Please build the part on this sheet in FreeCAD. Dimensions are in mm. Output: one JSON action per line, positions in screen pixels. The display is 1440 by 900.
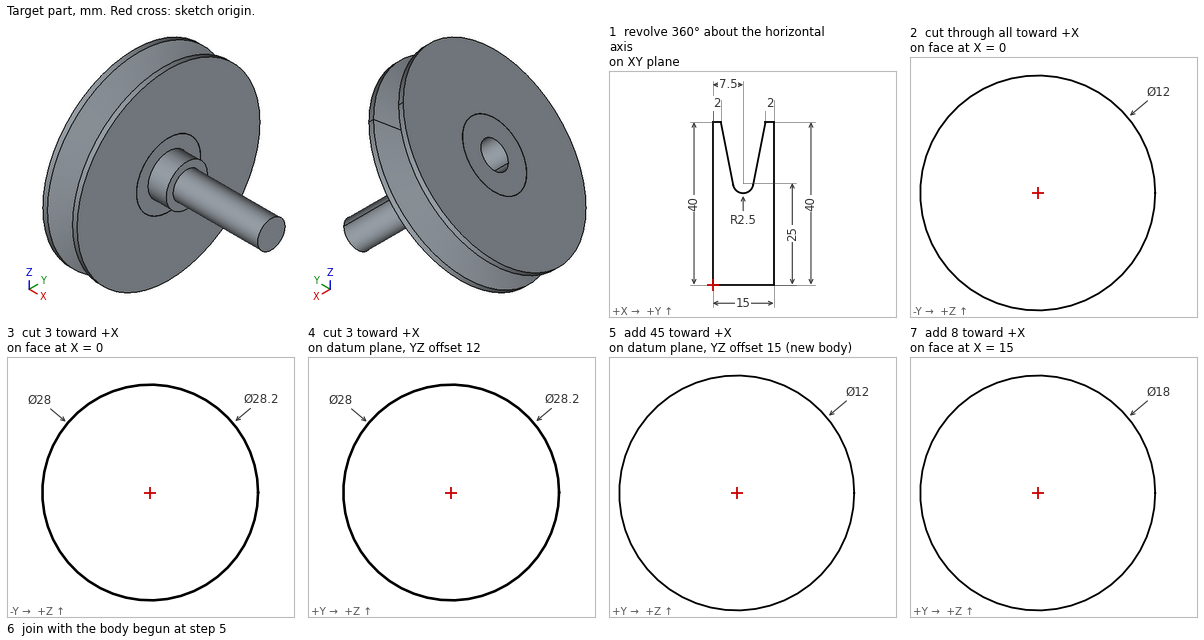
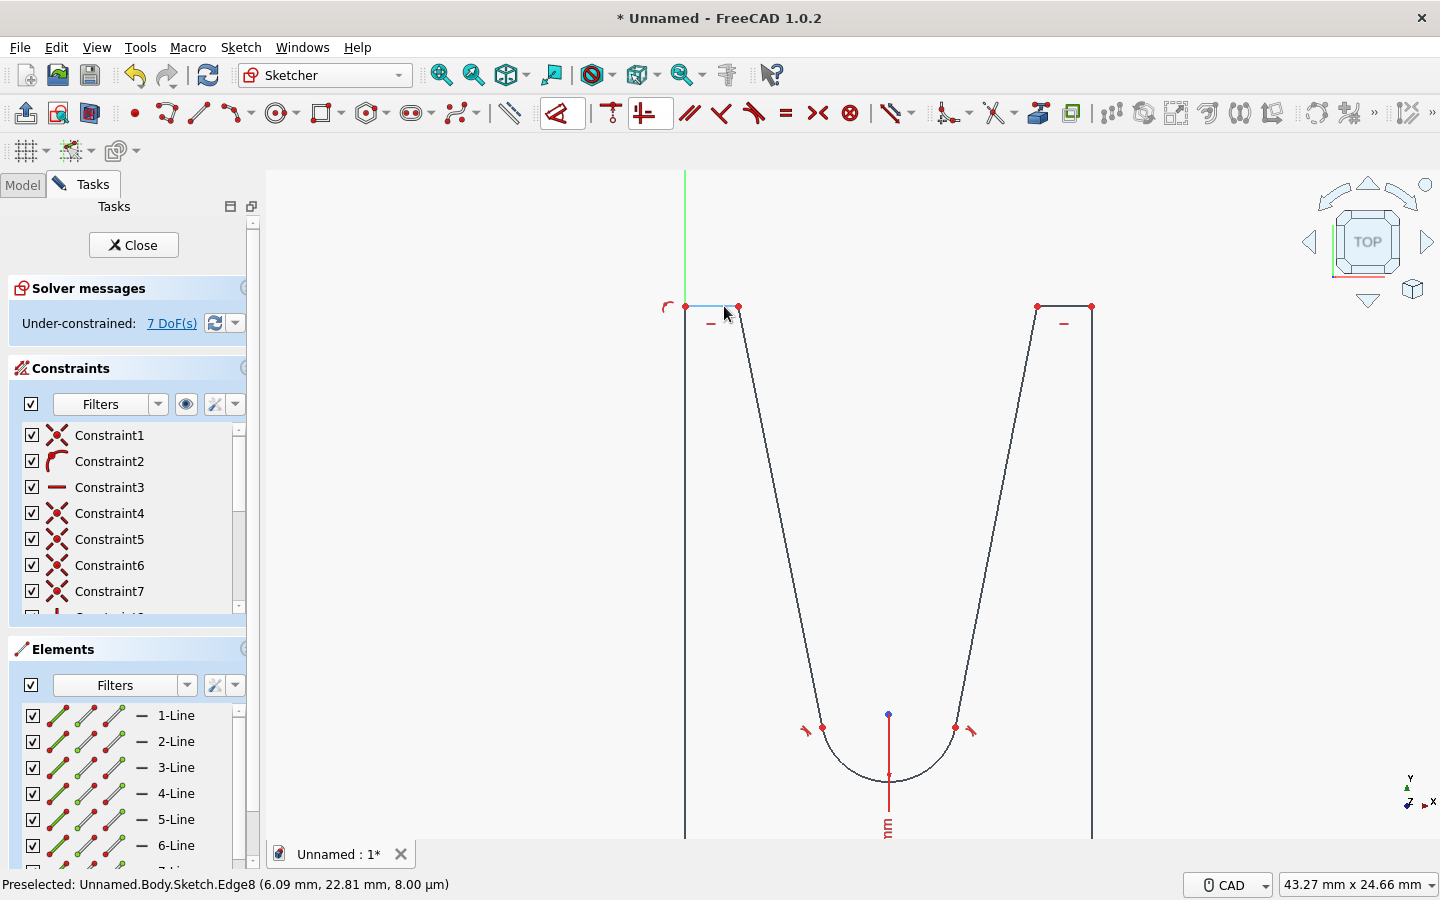
{"action": "left_click", "coordinate": [722, 306]}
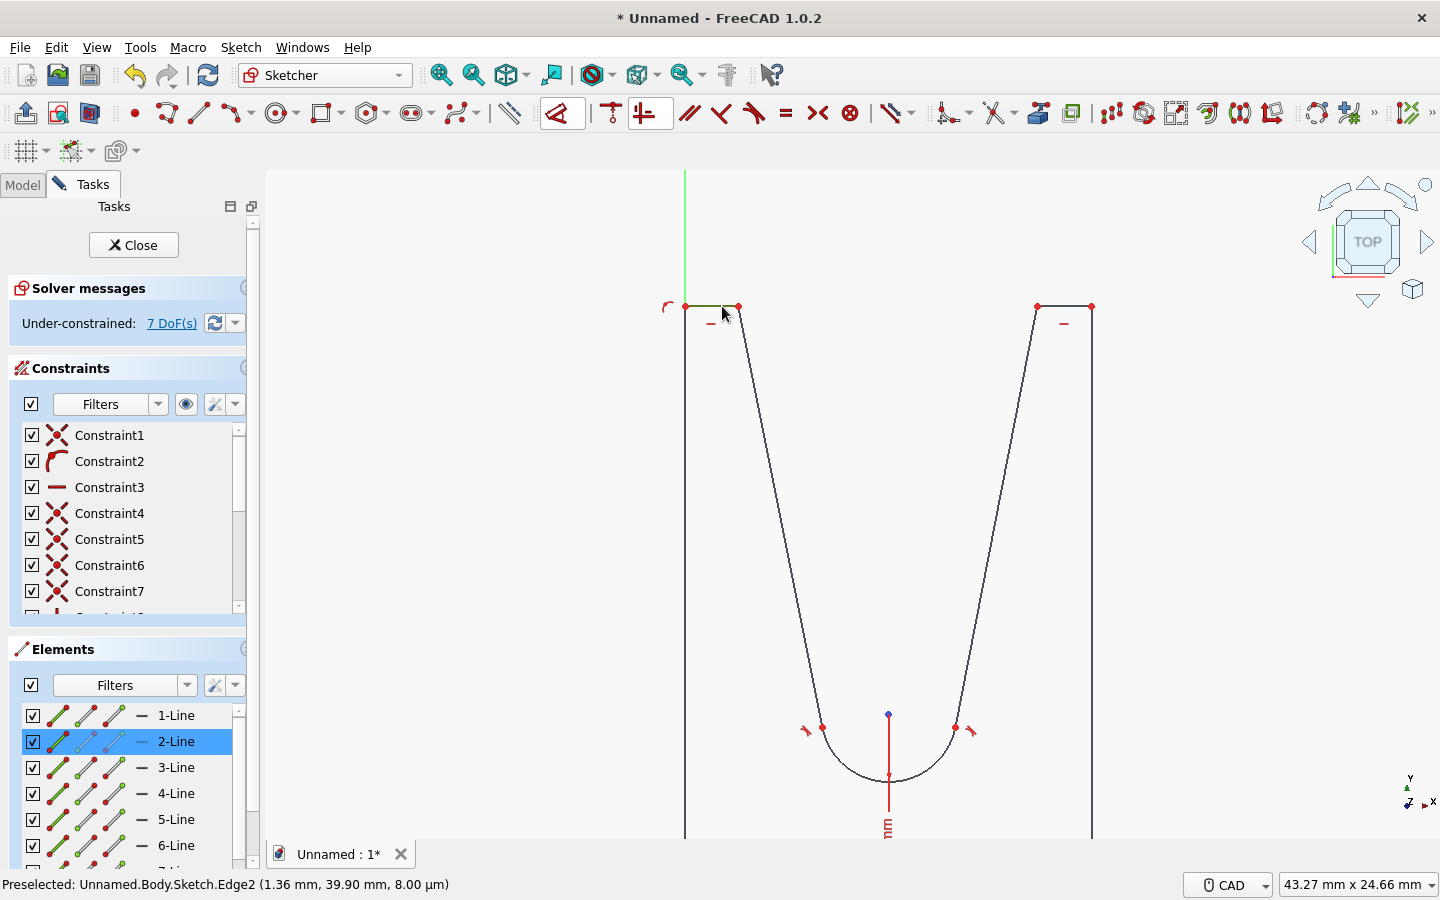
{"action": "key", "text": "l"}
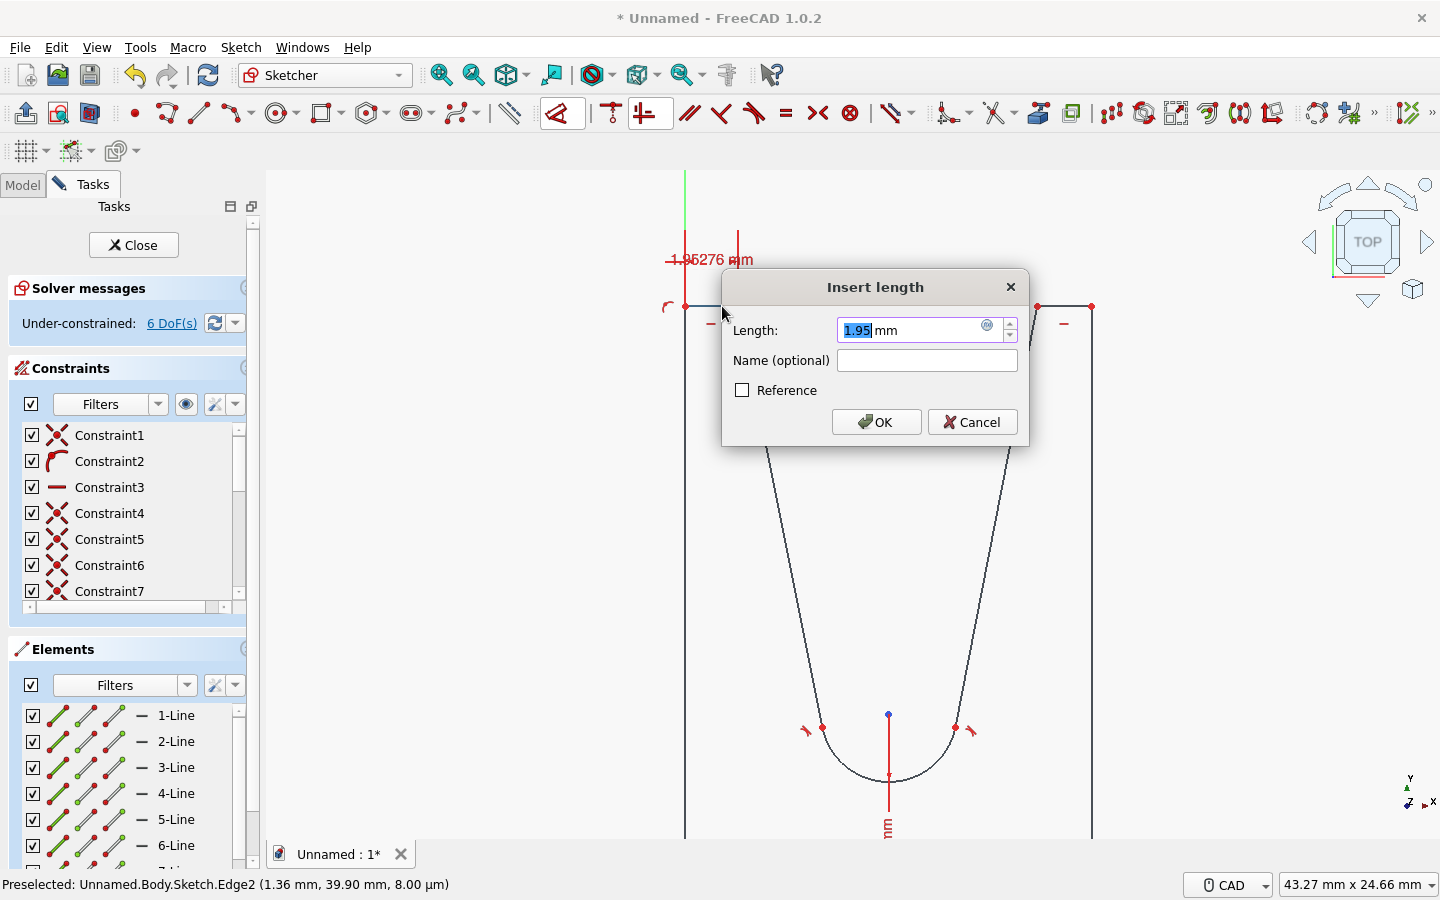
{"action": "type", "text": "2"}
{"action": "key", "text": "Return"}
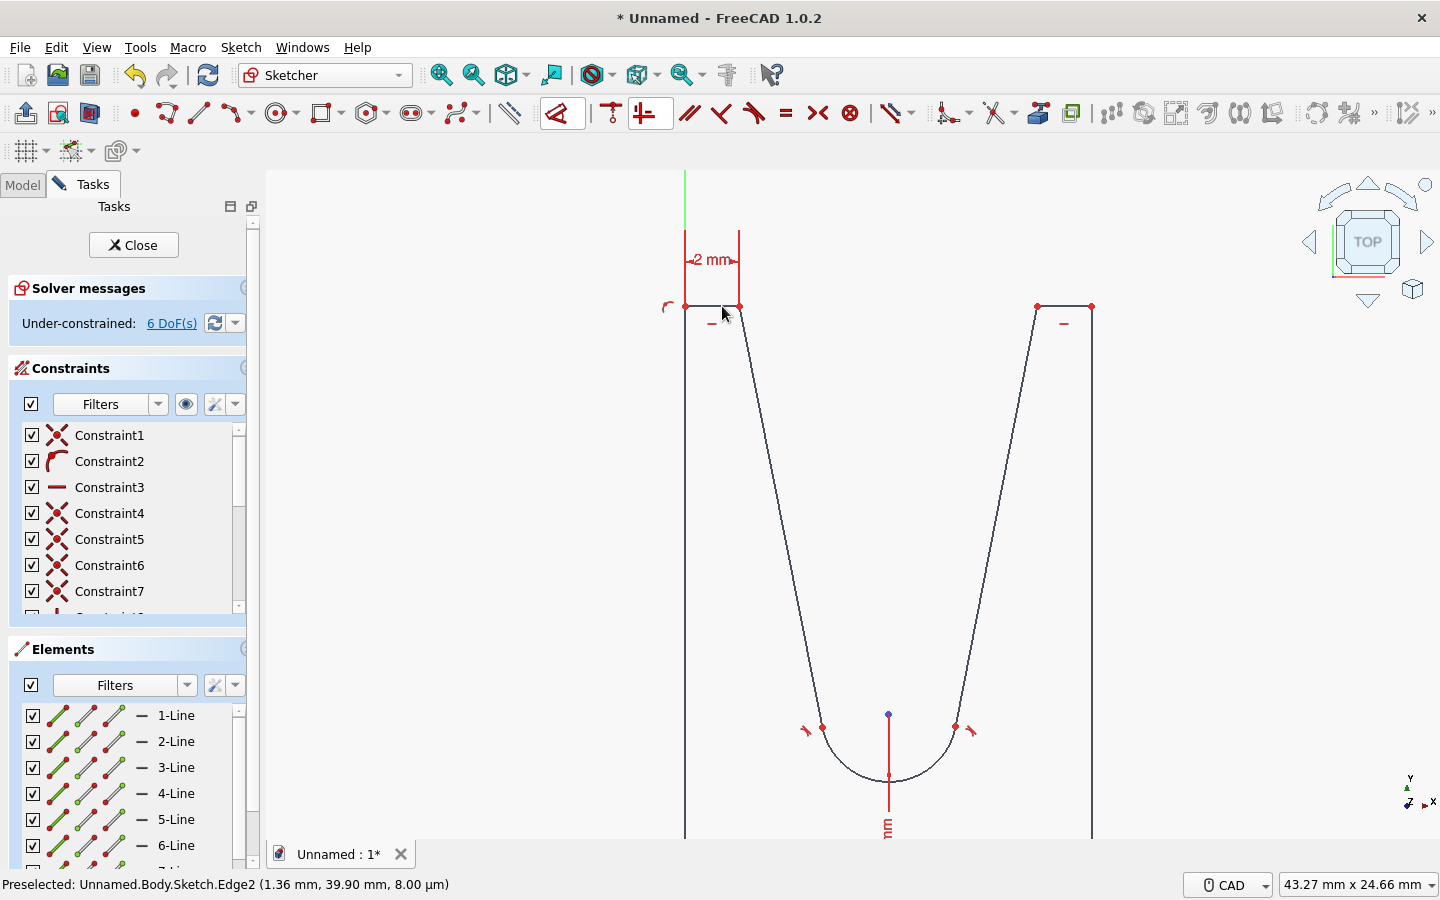
{"action": "left_click", "coordinate": [1075, 306]}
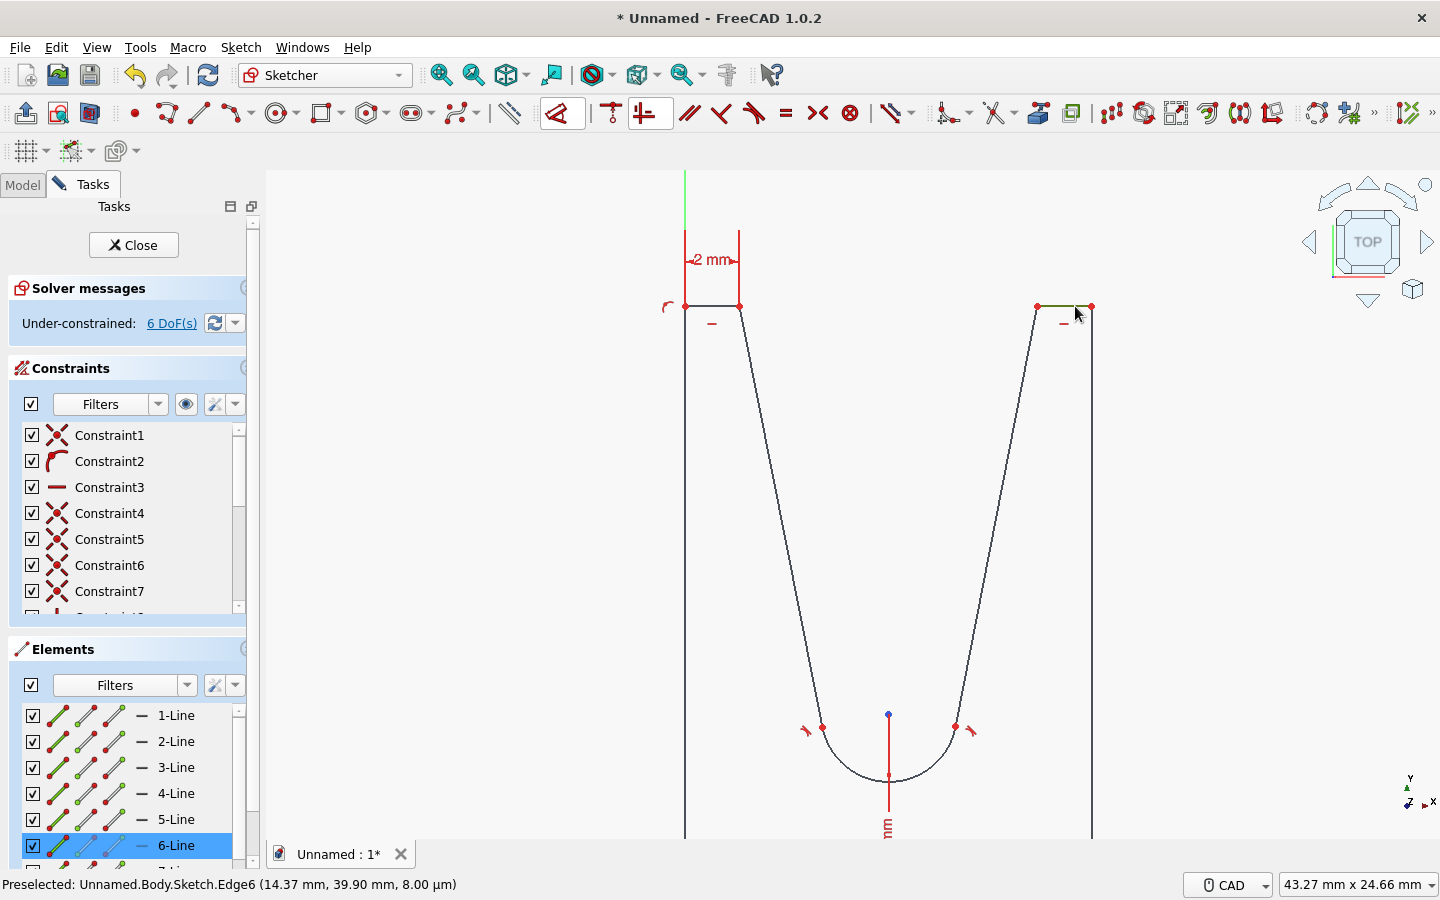
{"action": "left_click", "coordinate": [580, 114]}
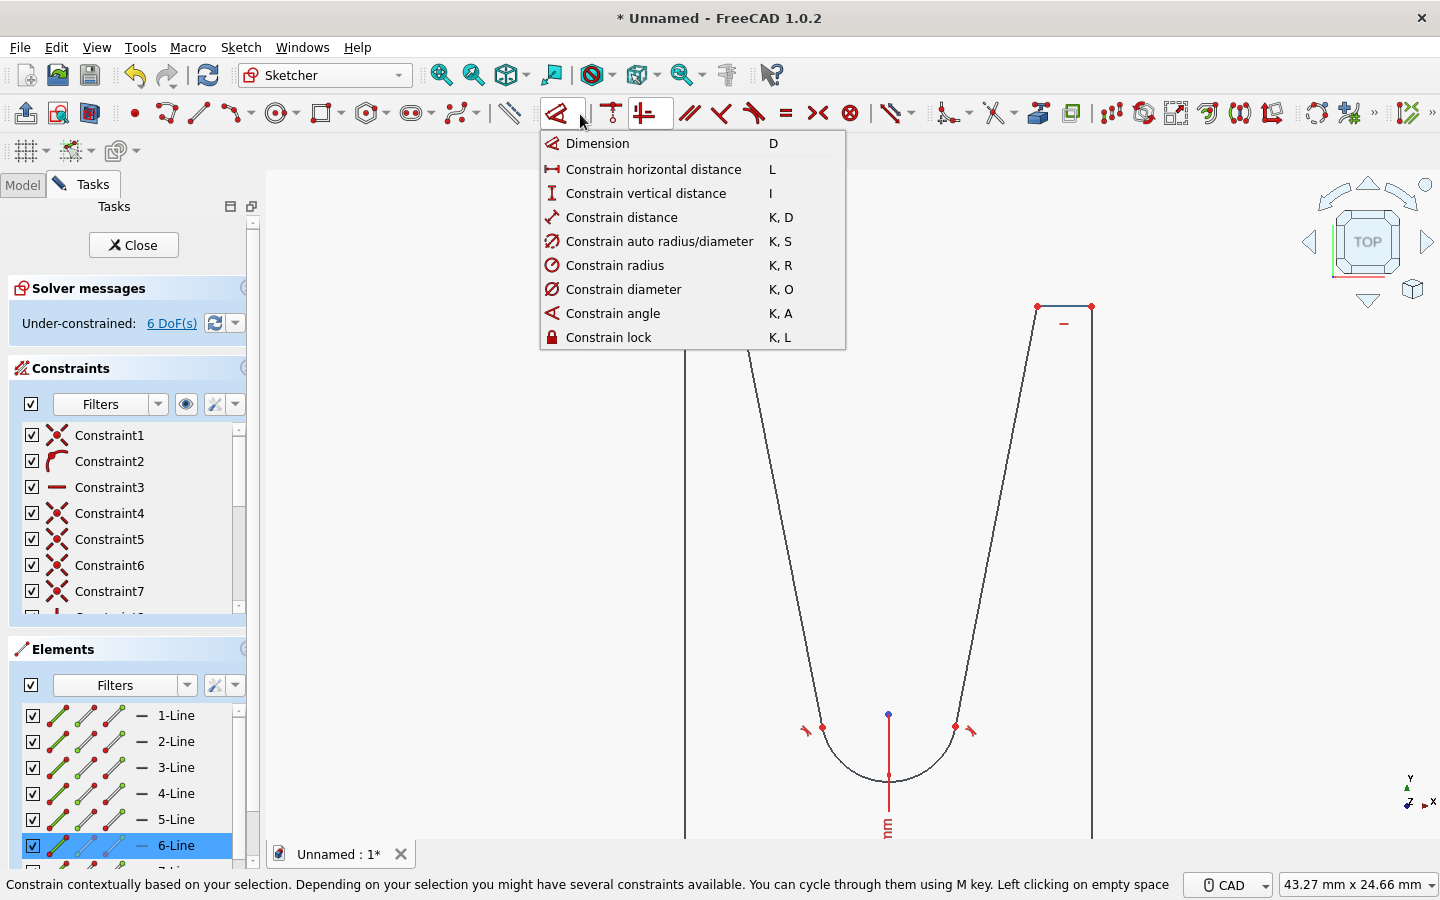
{"action": "left_click", "coordinate": [693, 169]}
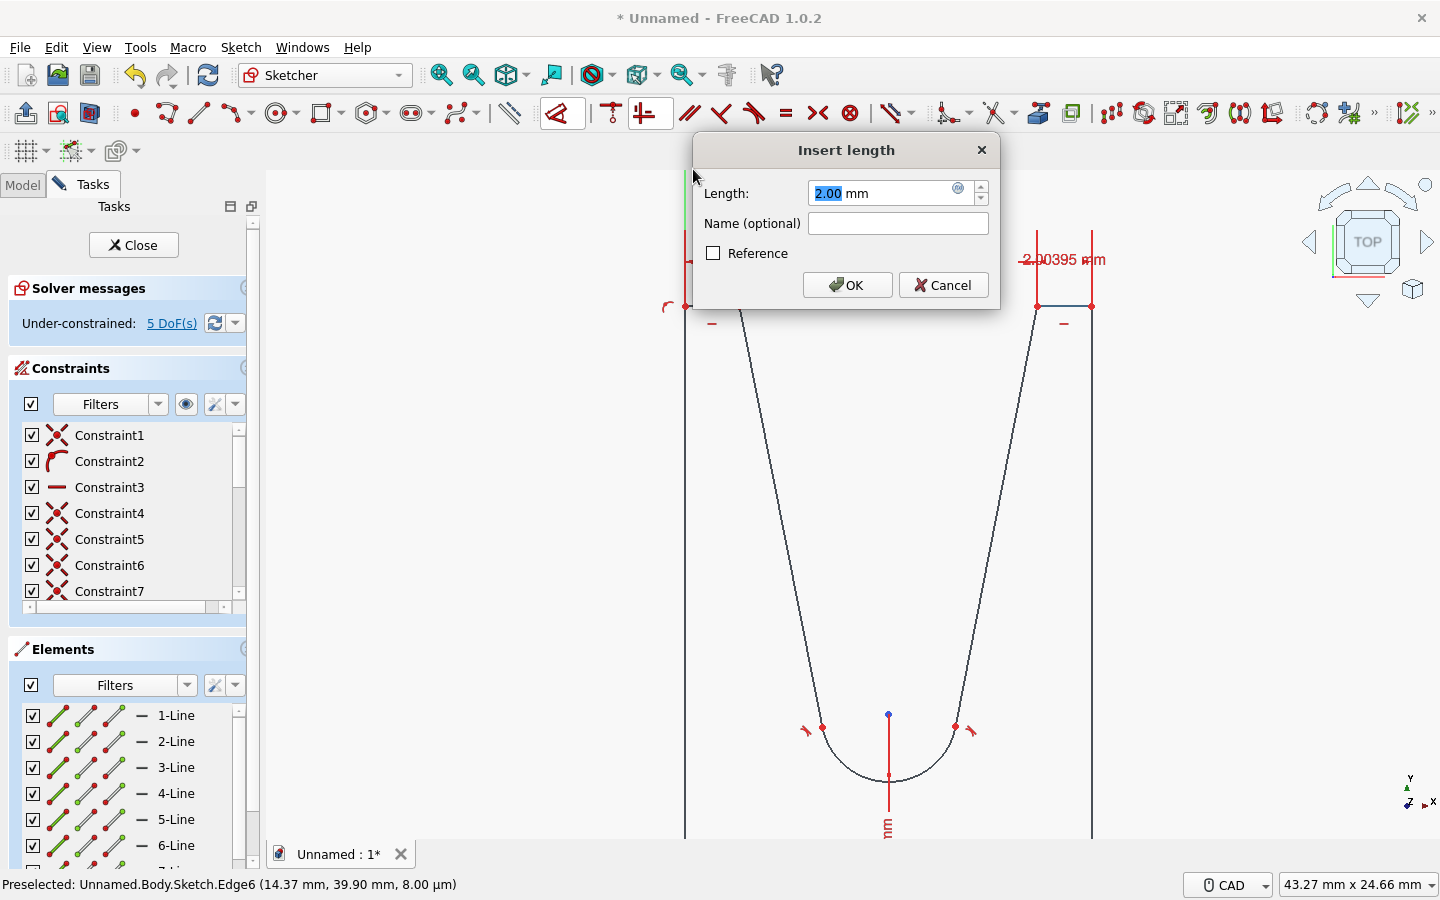
{"action": "type", "text": "2"}
{"action": "key", "text": "Return"}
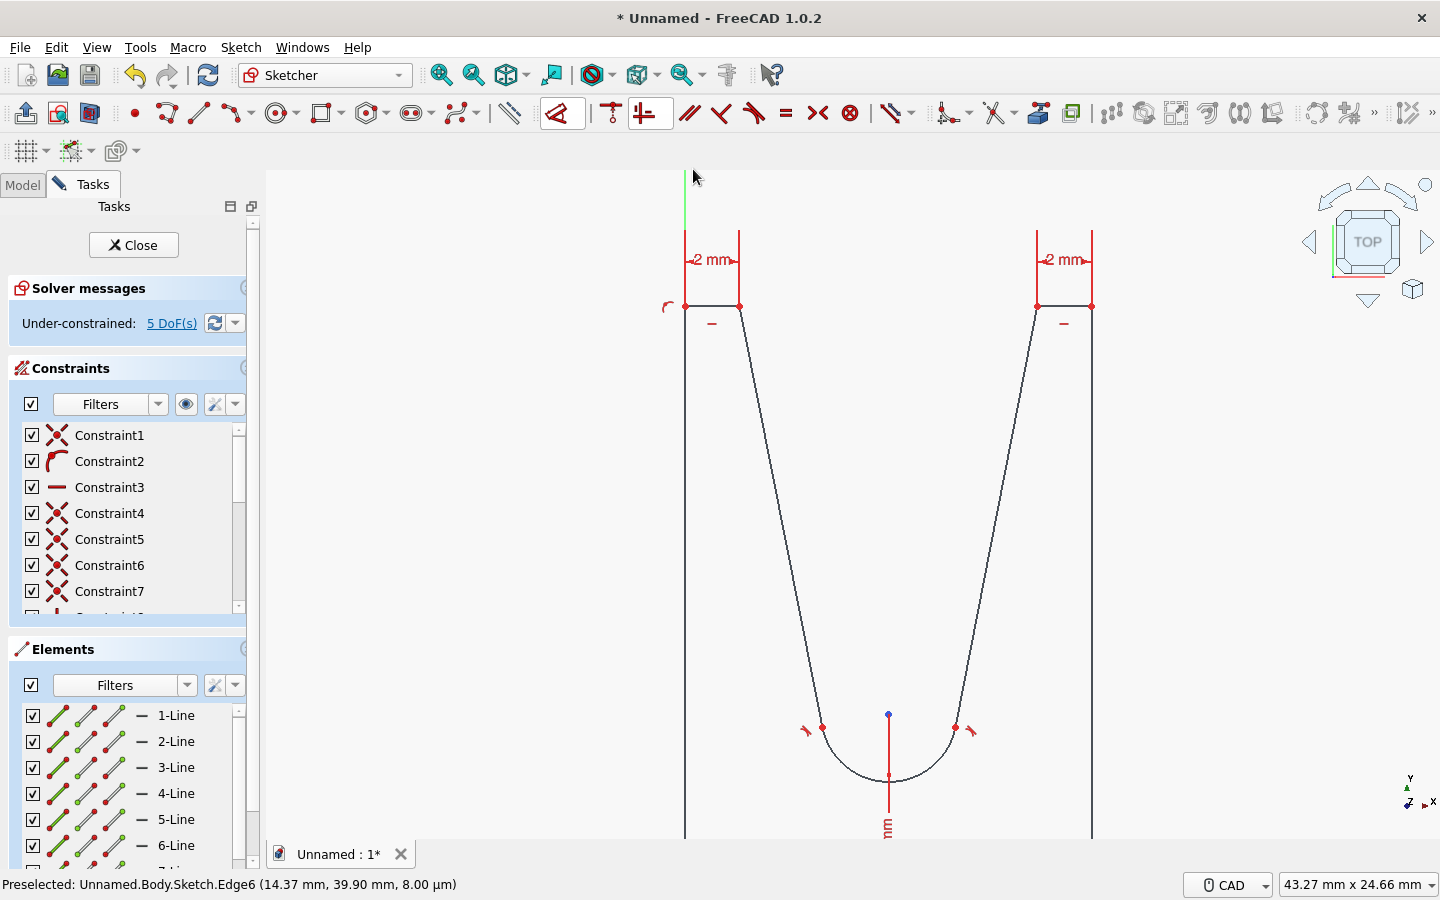
{"action": "left_click", "coordinate": [685, 631]}